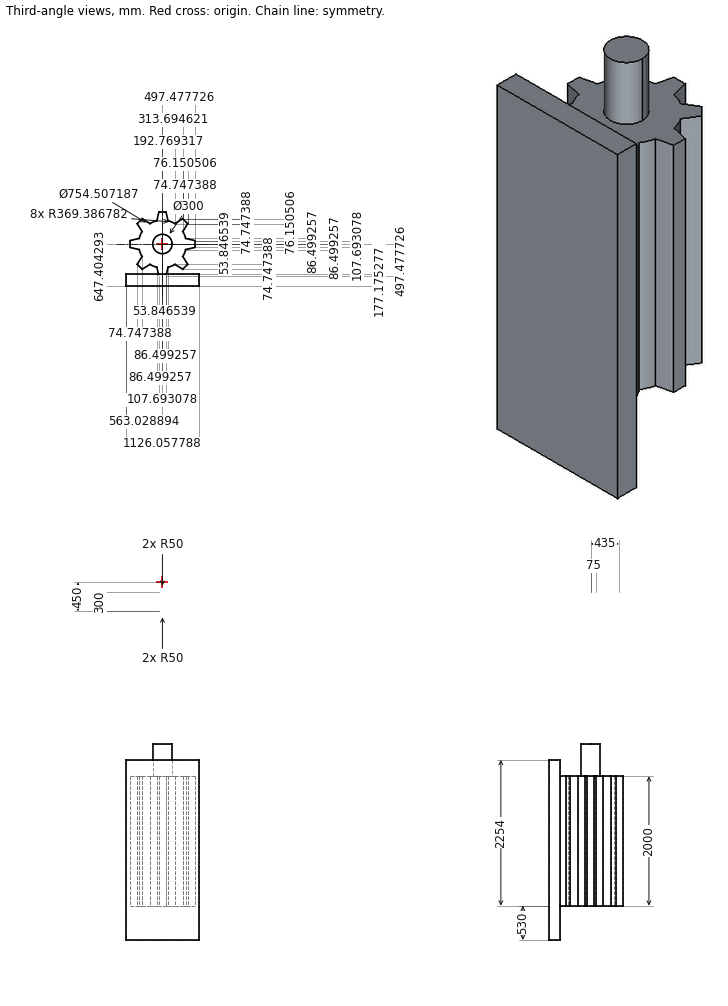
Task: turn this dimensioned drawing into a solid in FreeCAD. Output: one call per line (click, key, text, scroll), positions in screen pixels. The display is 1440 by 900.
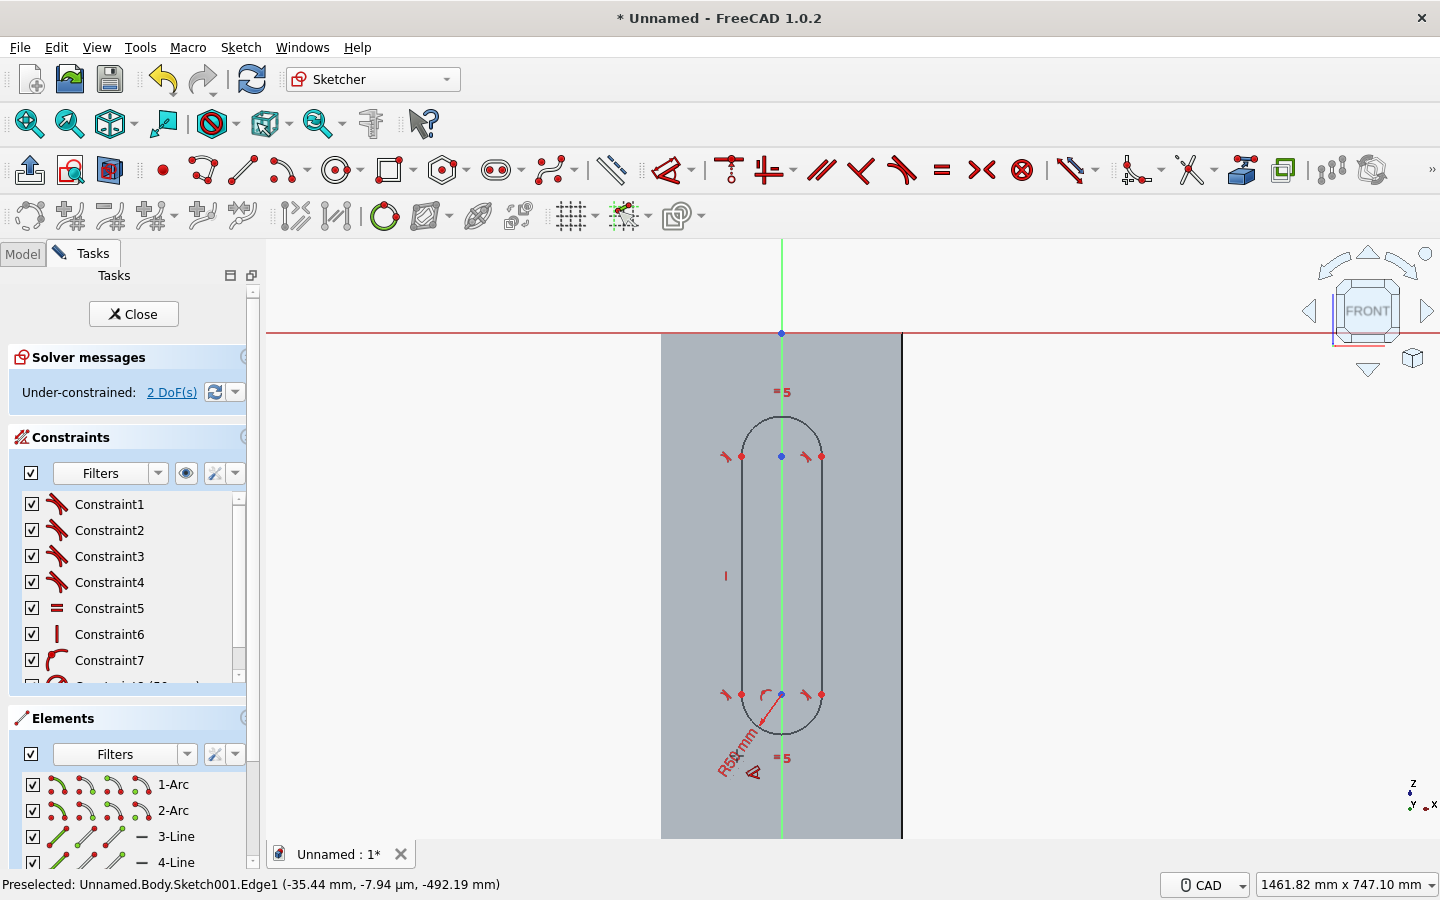
click(742, 623)
click(708, 576)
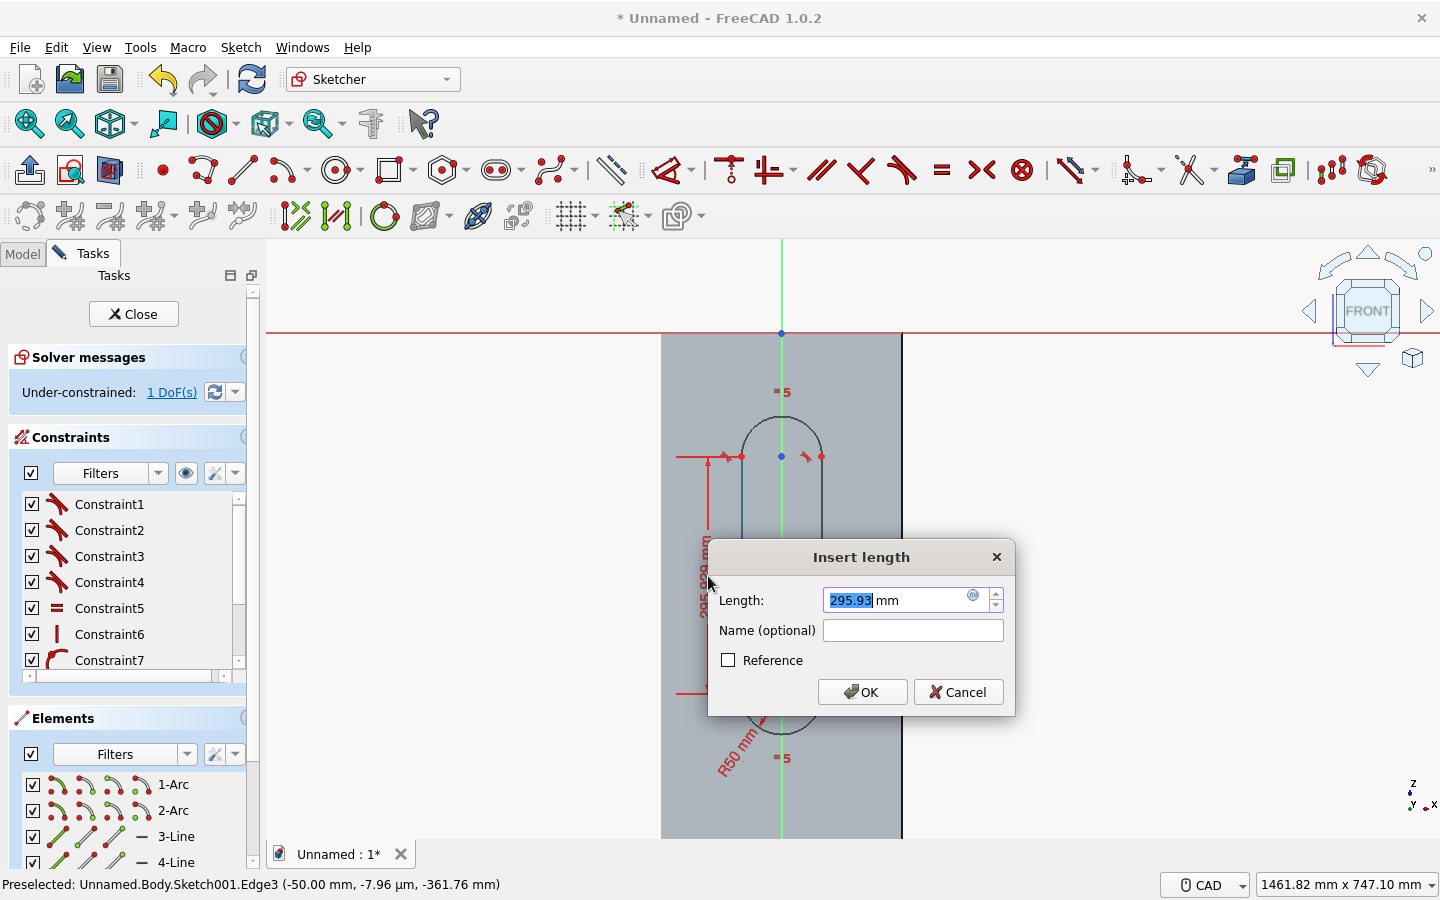
text(300)
key(Return)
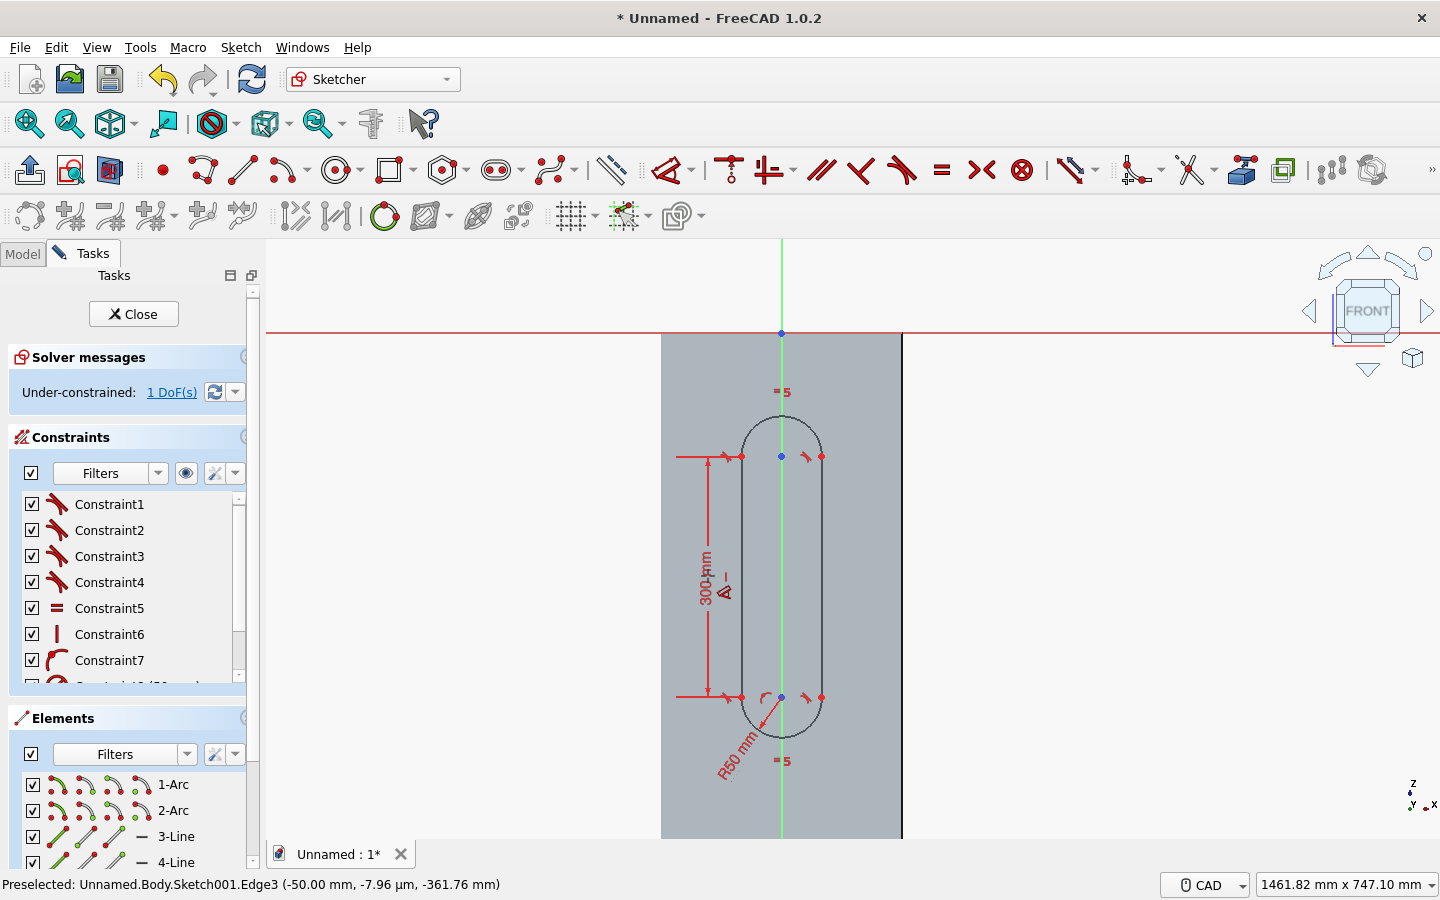
click(742, 697)
click(708, 515)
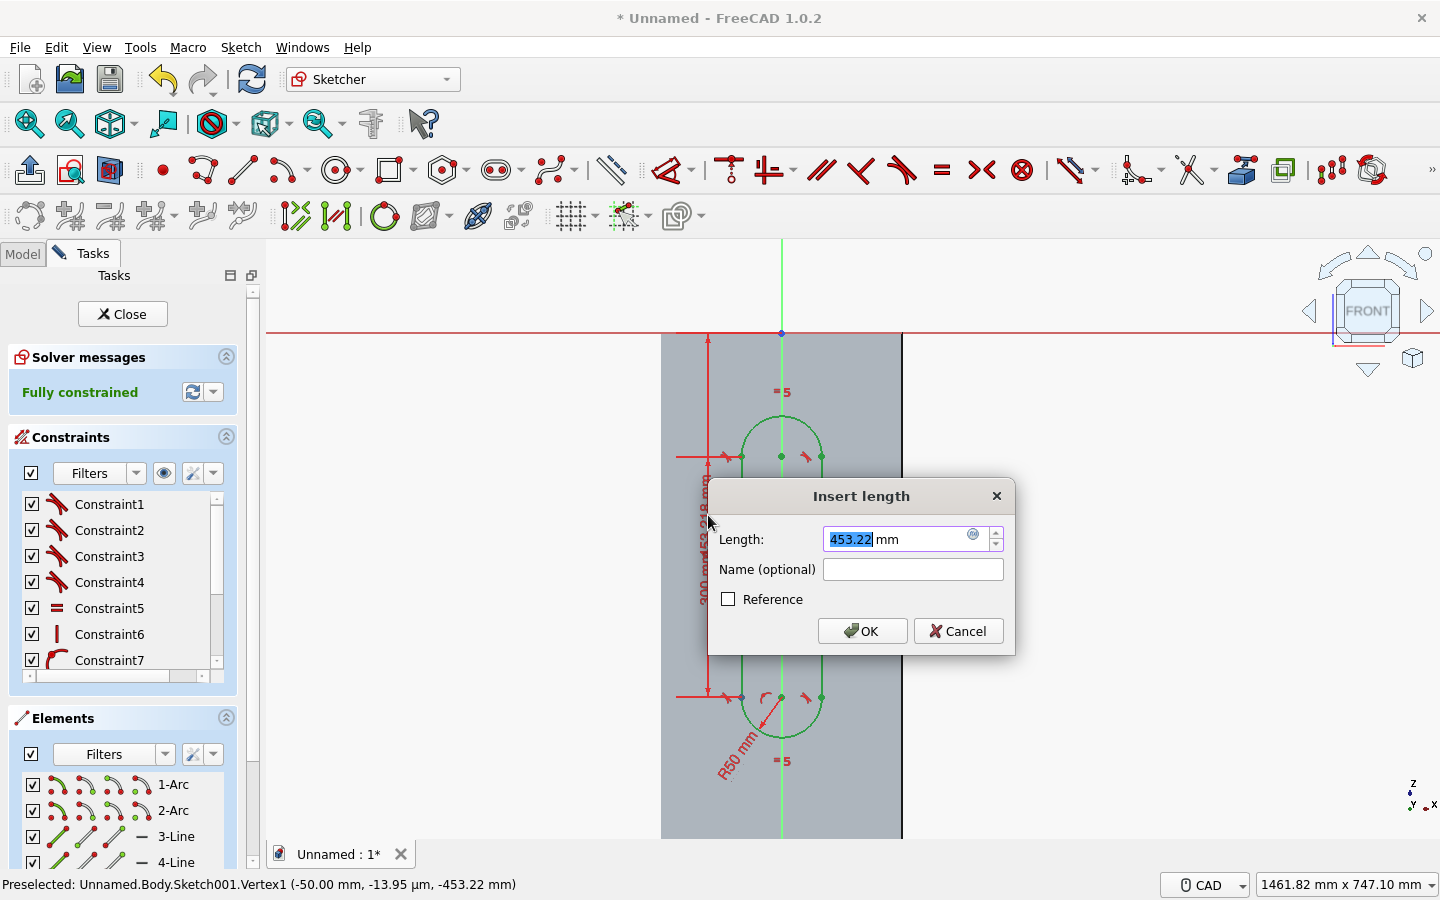
text(450)
key(Return)
key(Escape)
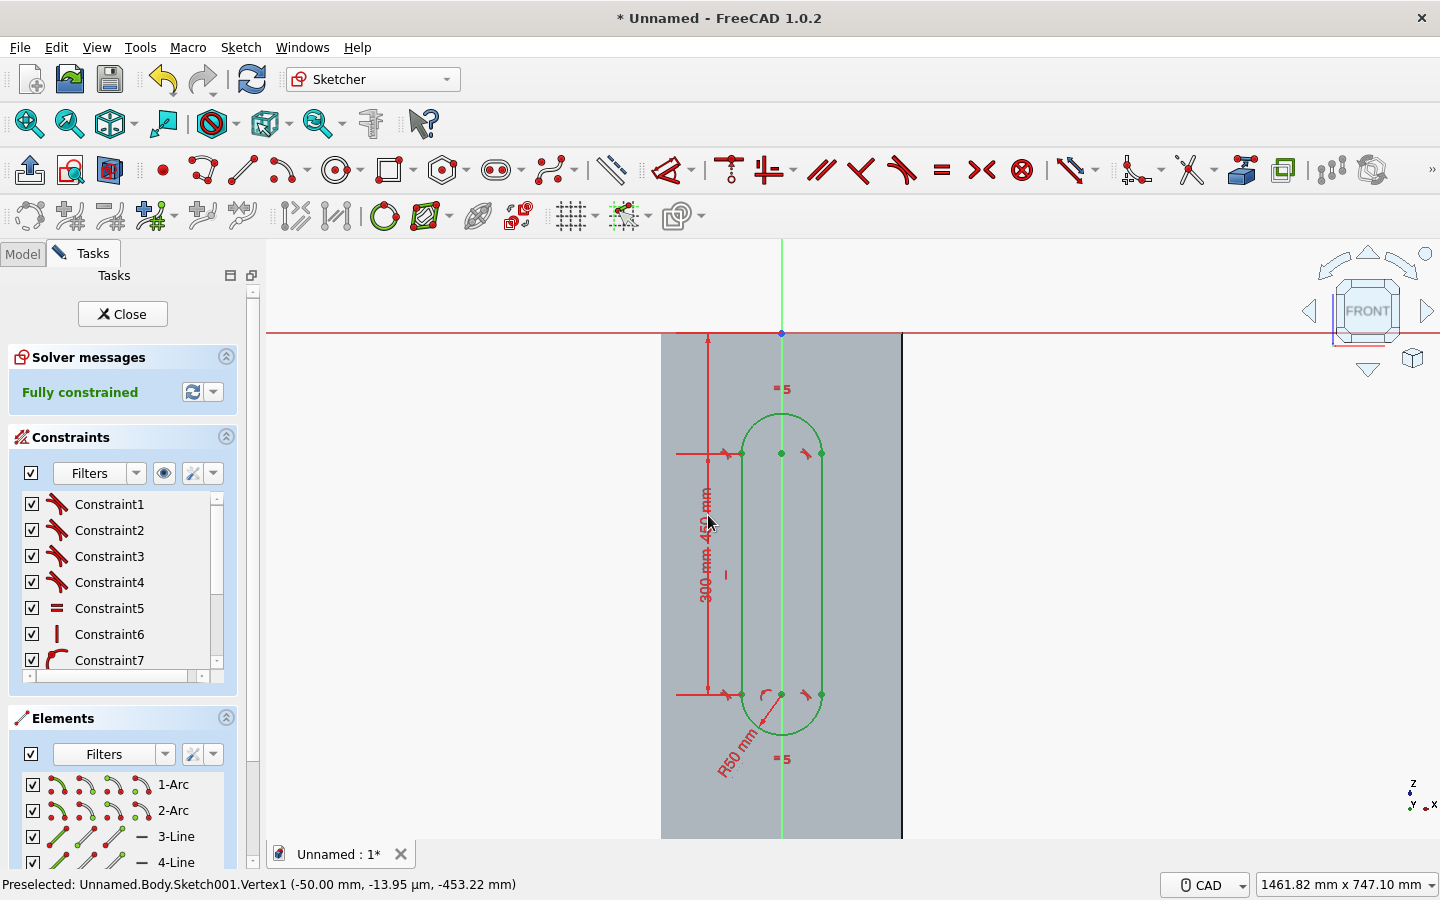
click(123, 314)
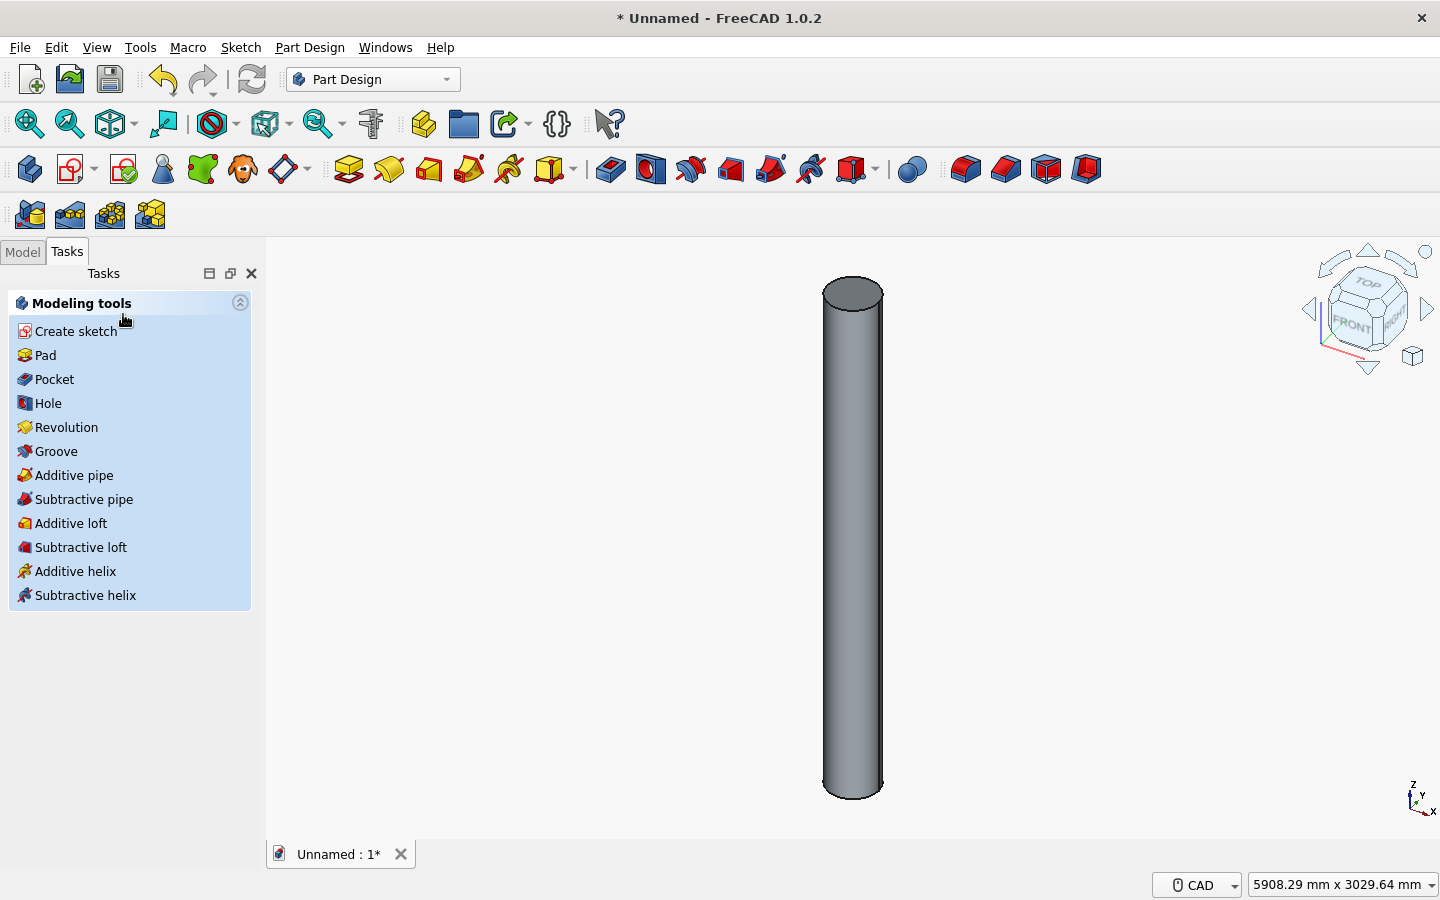
click(612, 170)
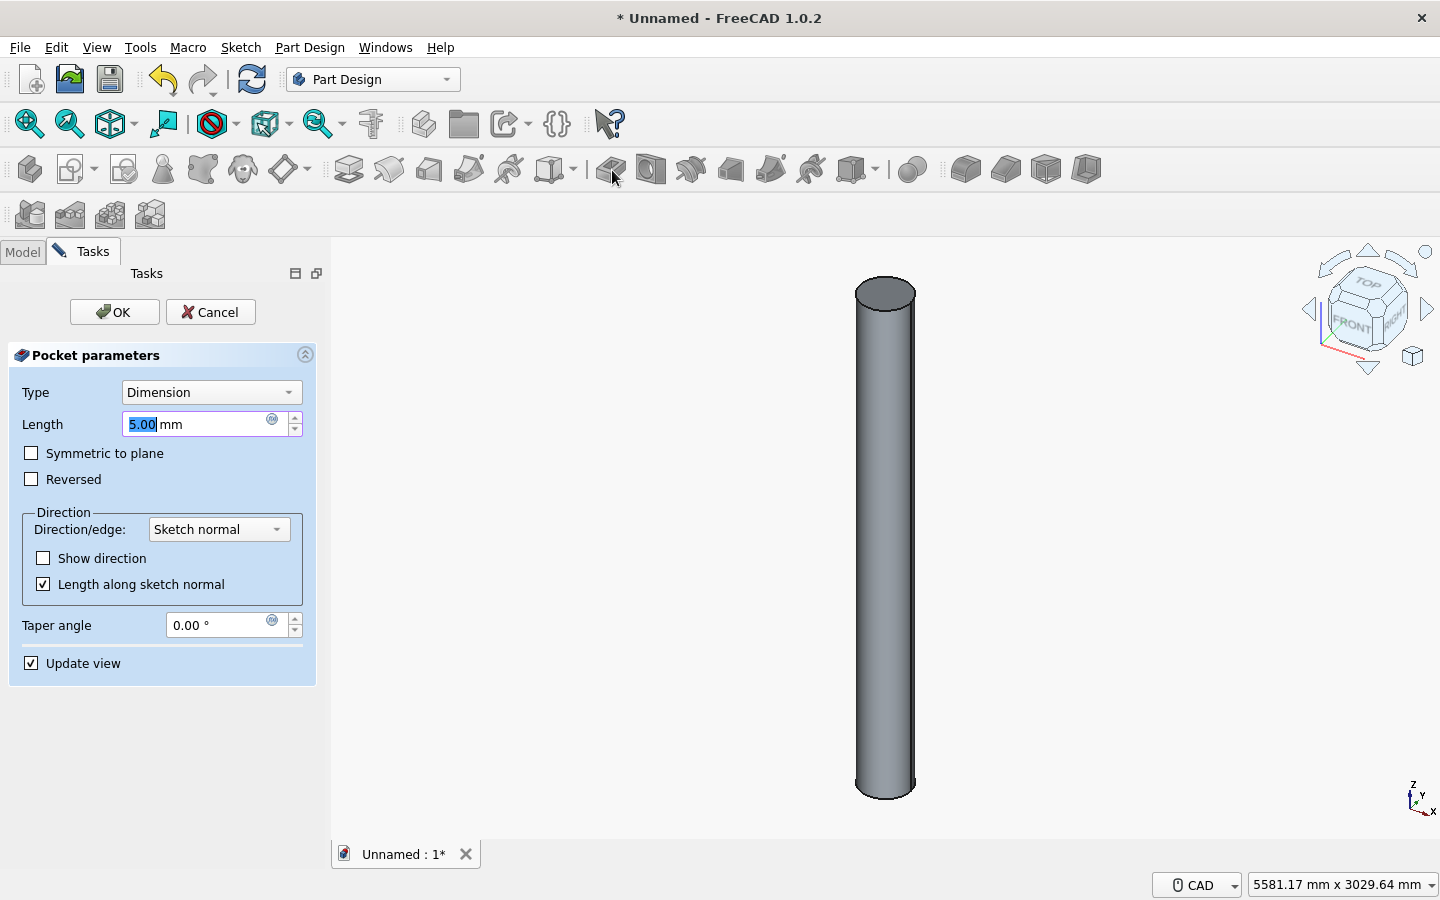
text(435)
key(Tab)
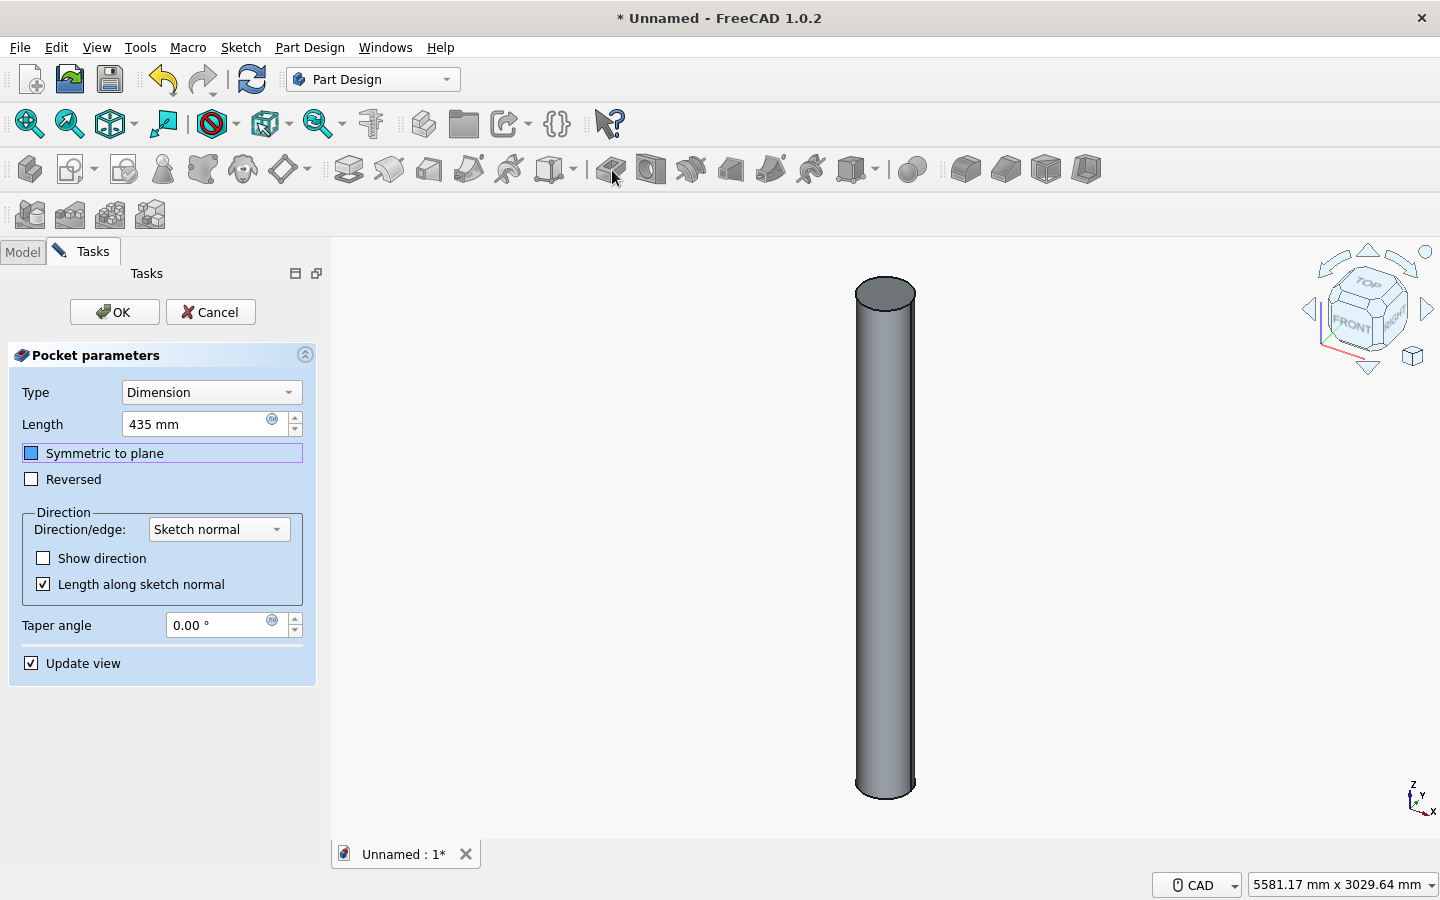
click(115, 312)